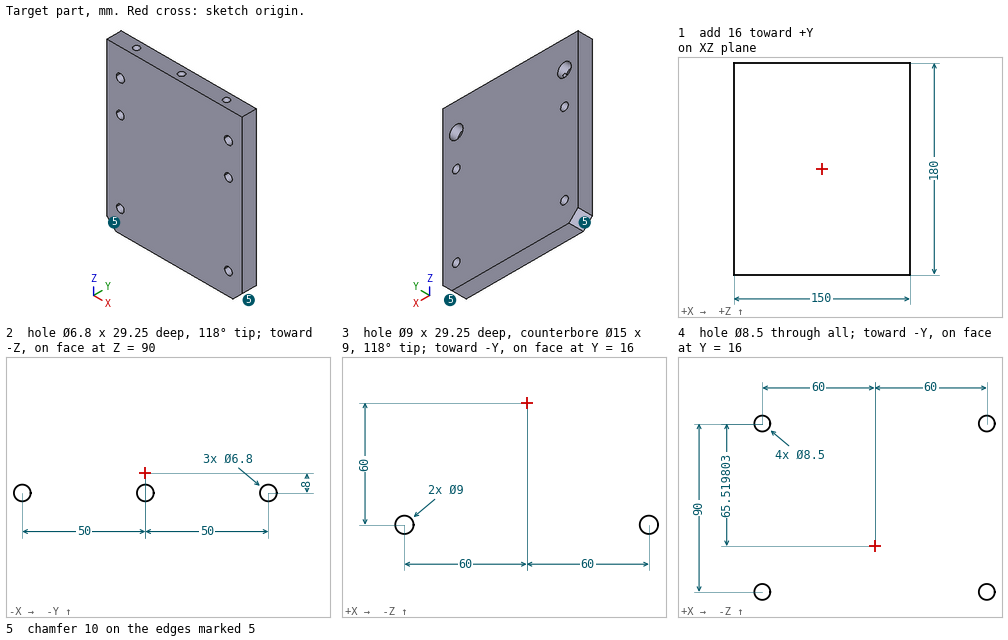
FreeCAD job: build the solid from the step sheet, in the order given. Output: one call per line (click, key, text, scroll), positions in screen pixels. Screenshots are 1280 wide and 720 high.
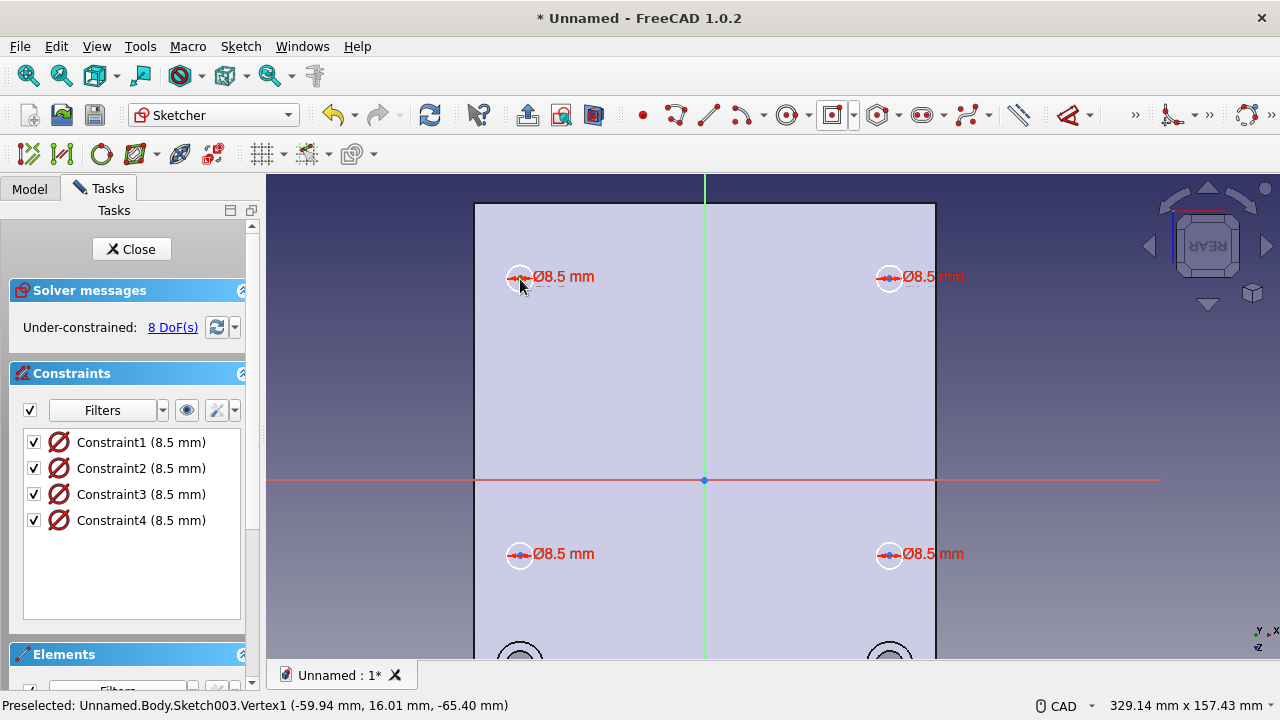
click(890, 279)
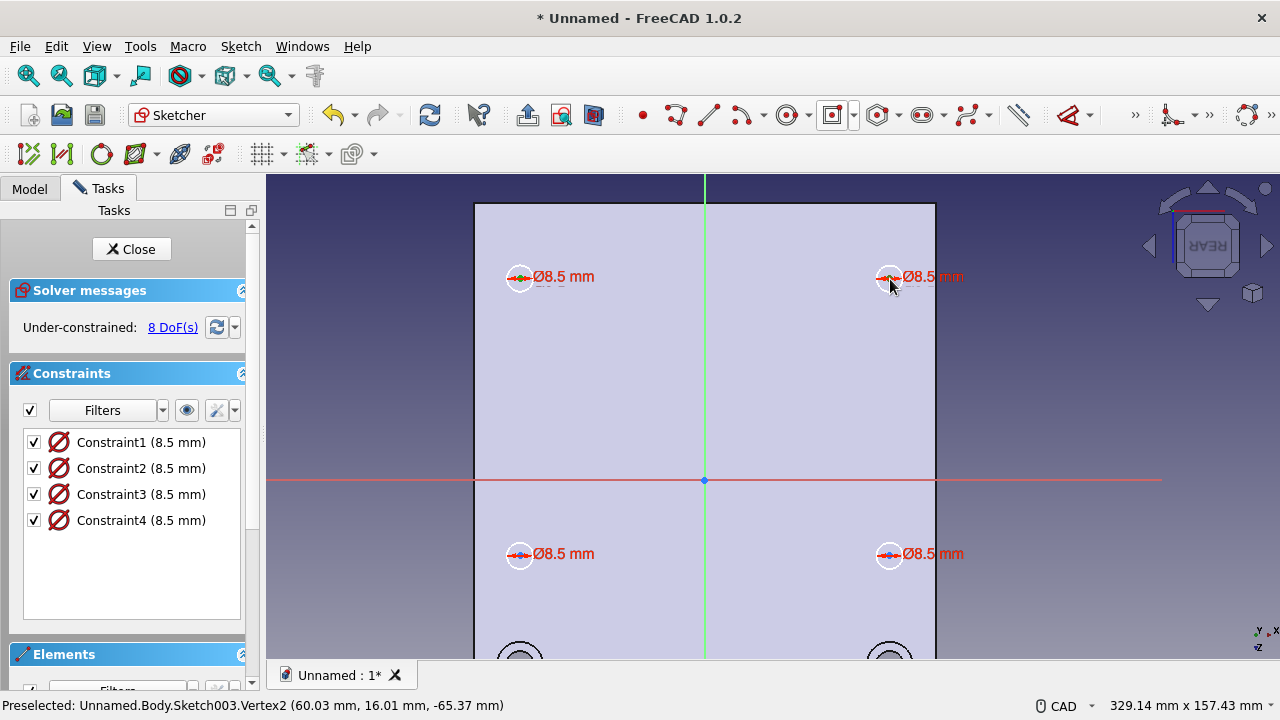
key(h)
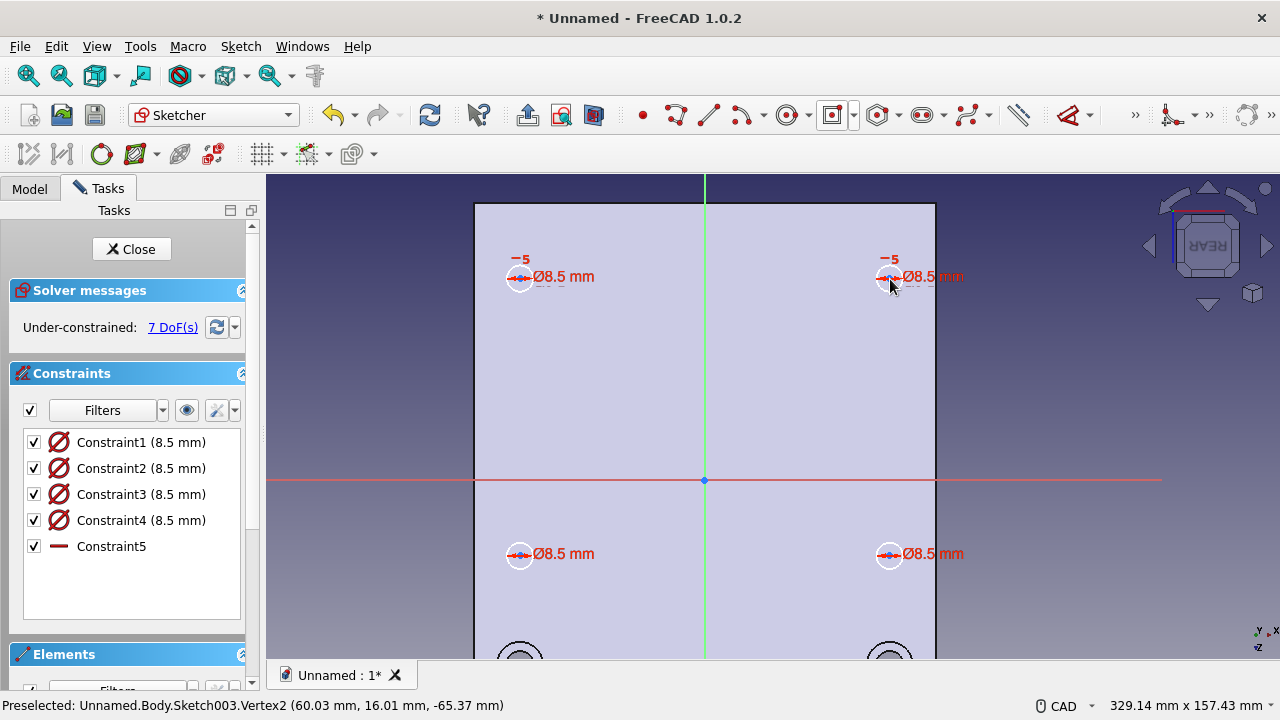
click(520, 279)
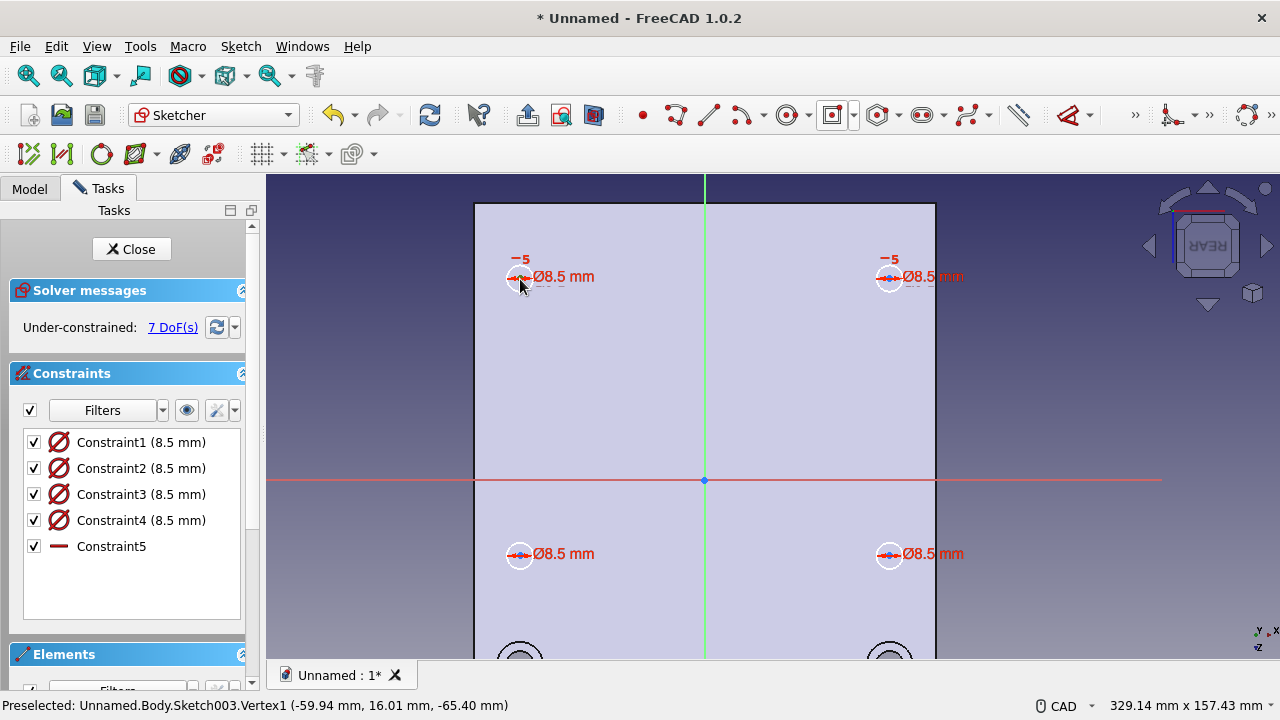
click(520, 556)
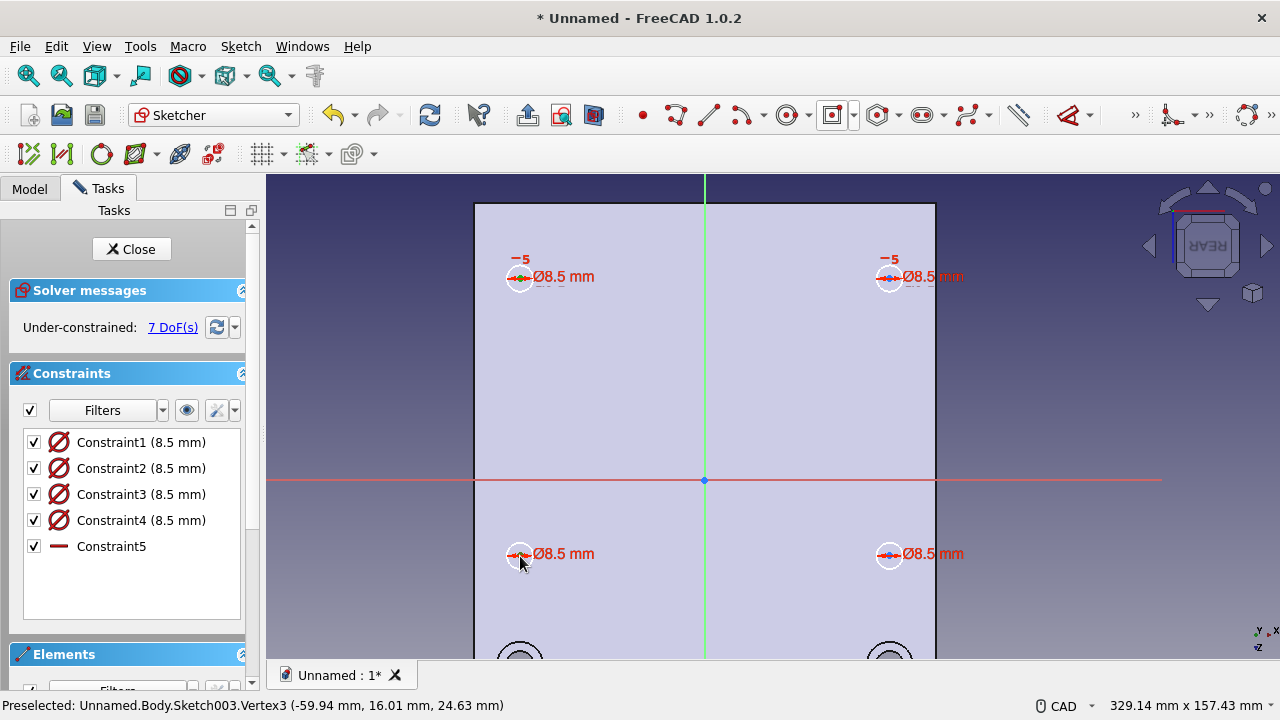
key(v)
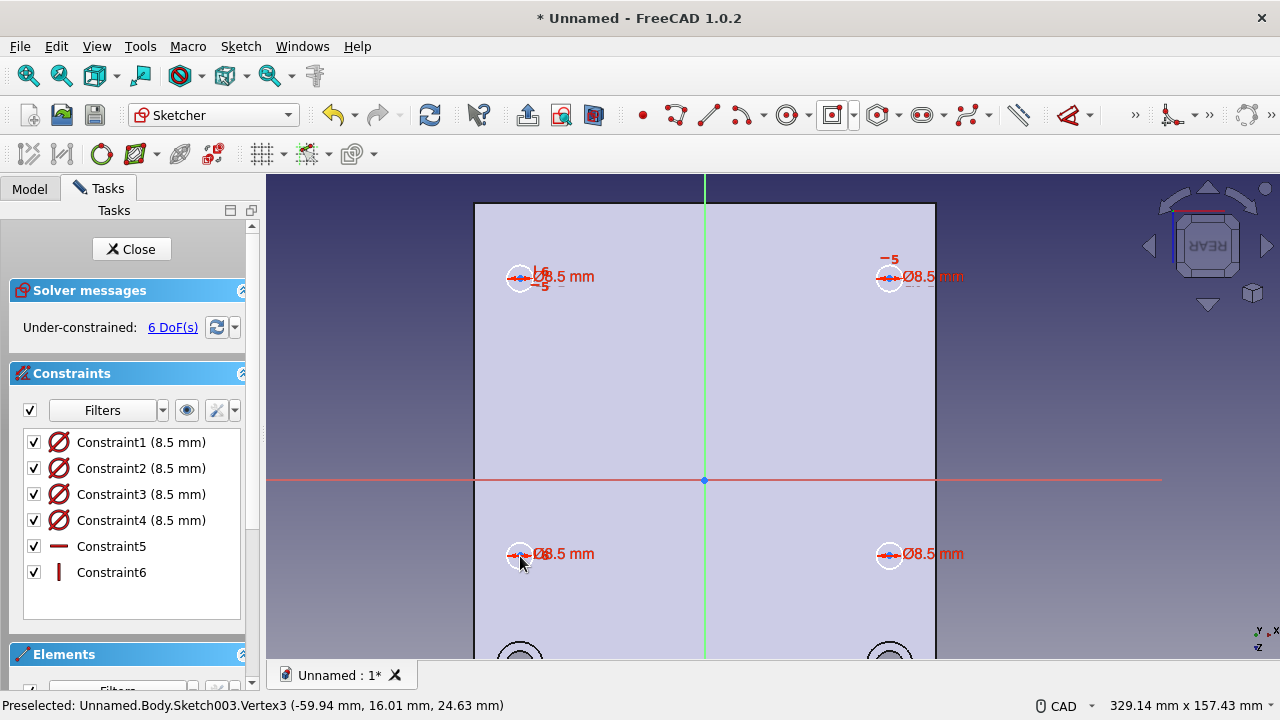
click(890, 279)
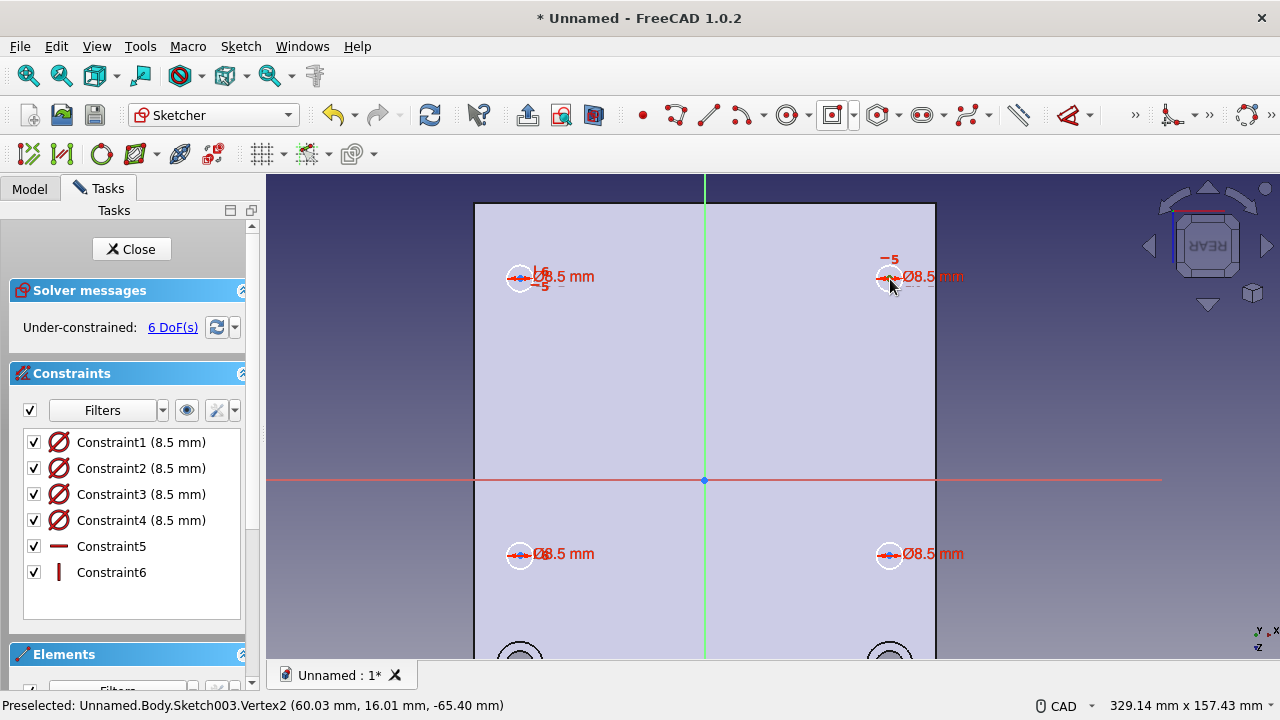
click(890, 556)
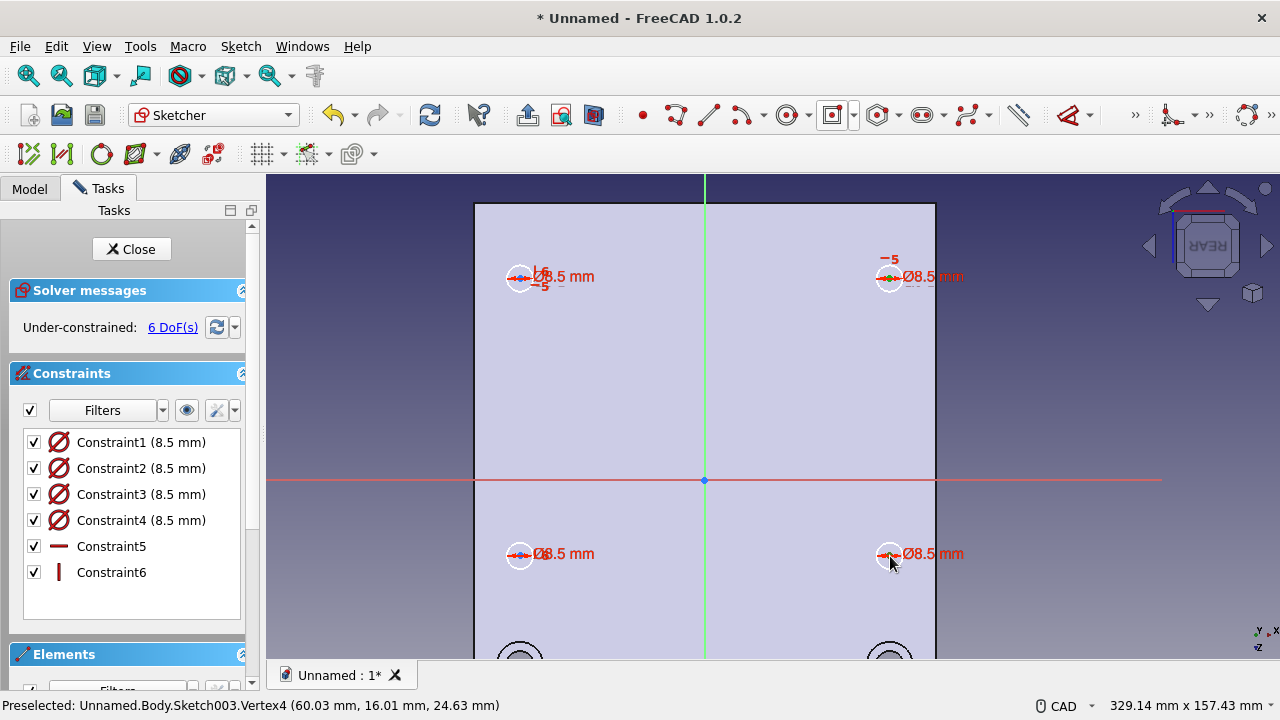
key(v)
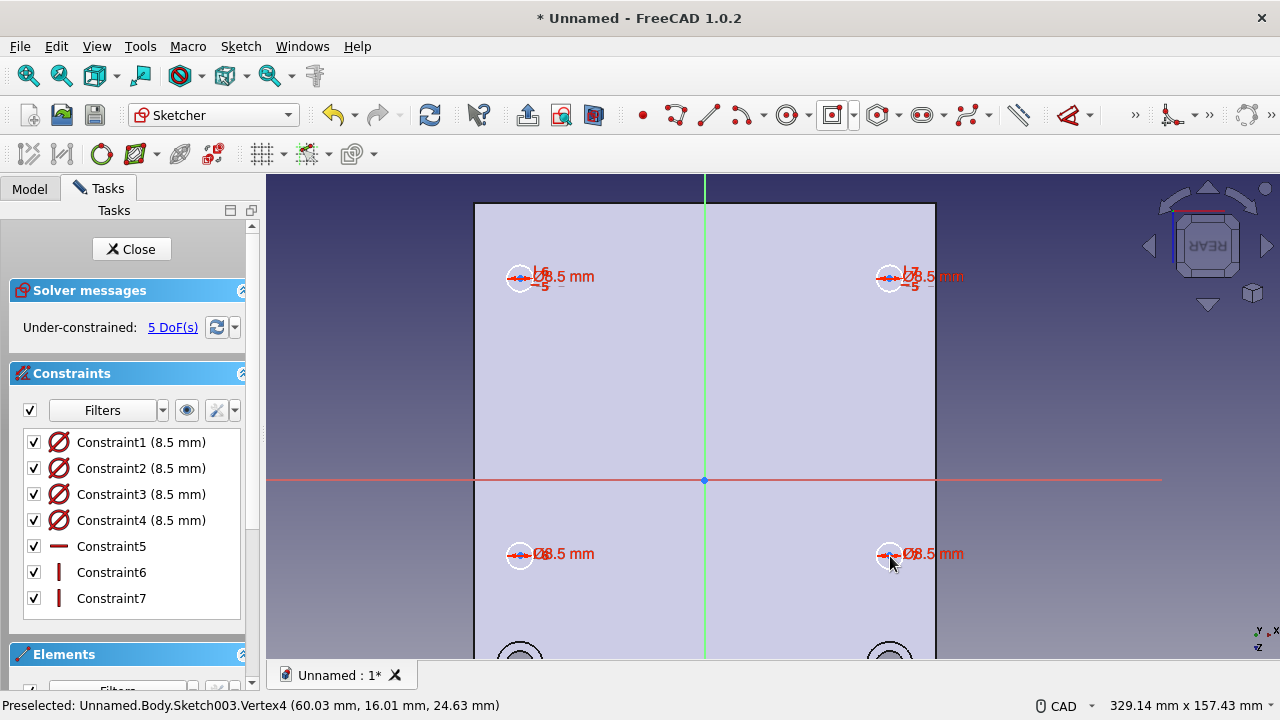
click(520, 556)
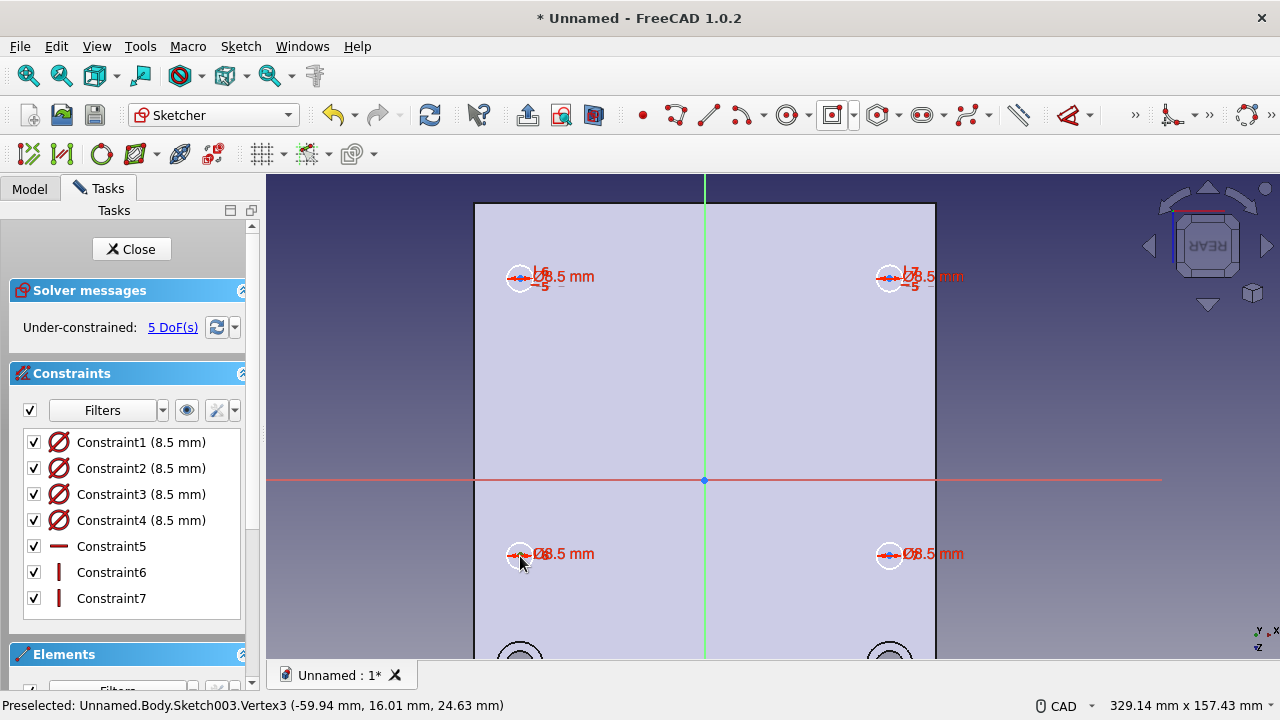
click(890, 556)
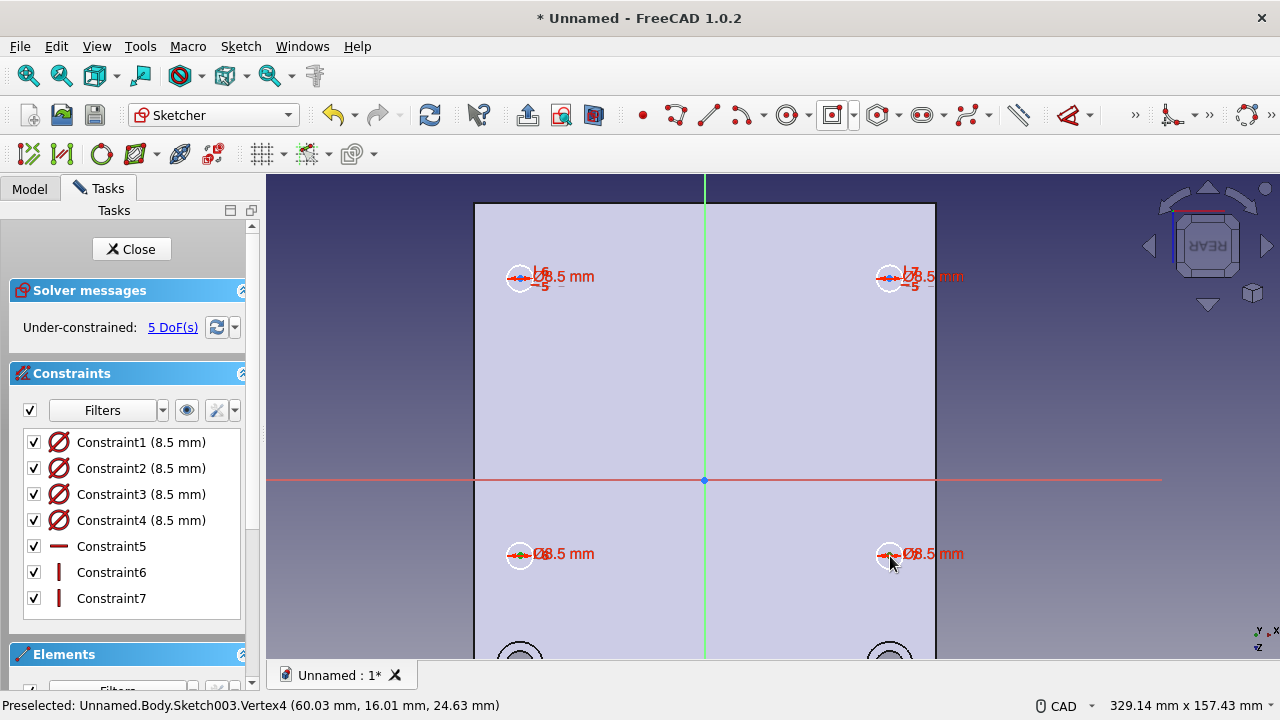
key(h)